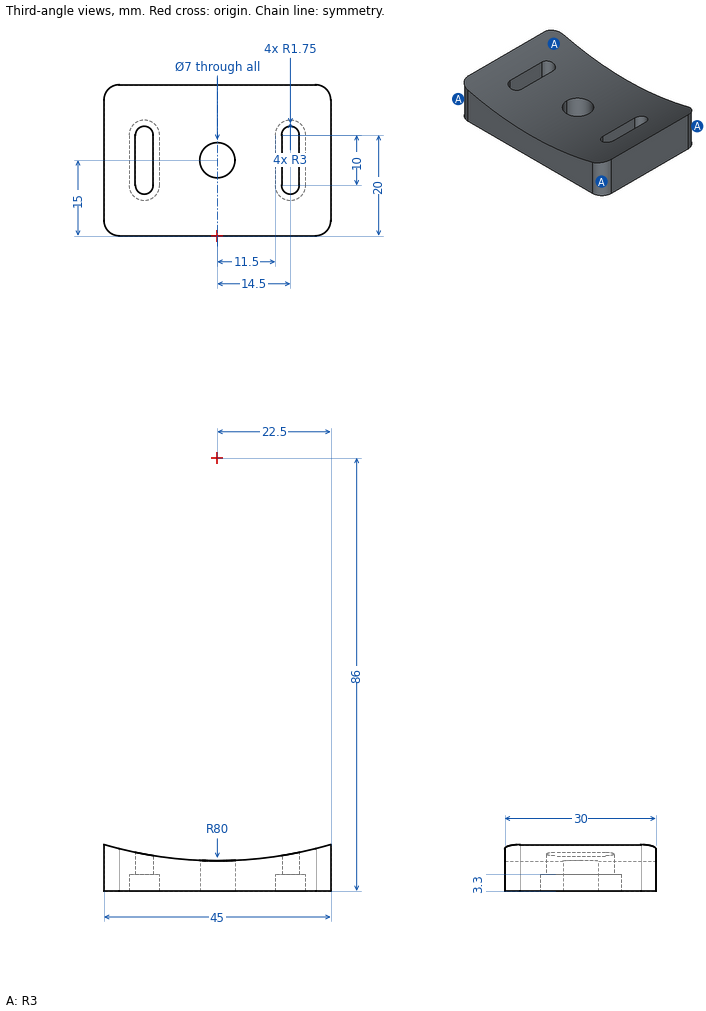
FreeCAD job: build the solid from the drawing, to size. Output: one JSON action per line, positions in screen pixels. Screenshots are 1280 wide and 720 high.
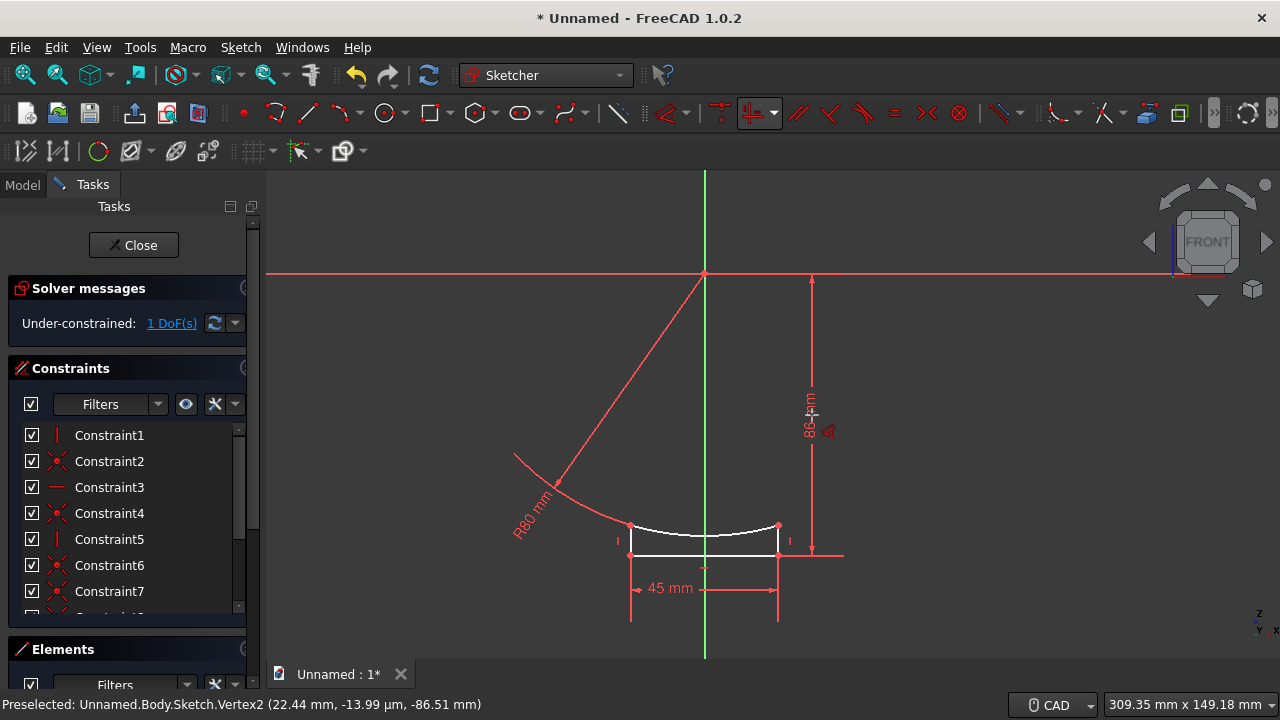
{"action": "left_click", "coordinate": [778, 525]}
{"action": "left_click", "coordinate": [742, 240]}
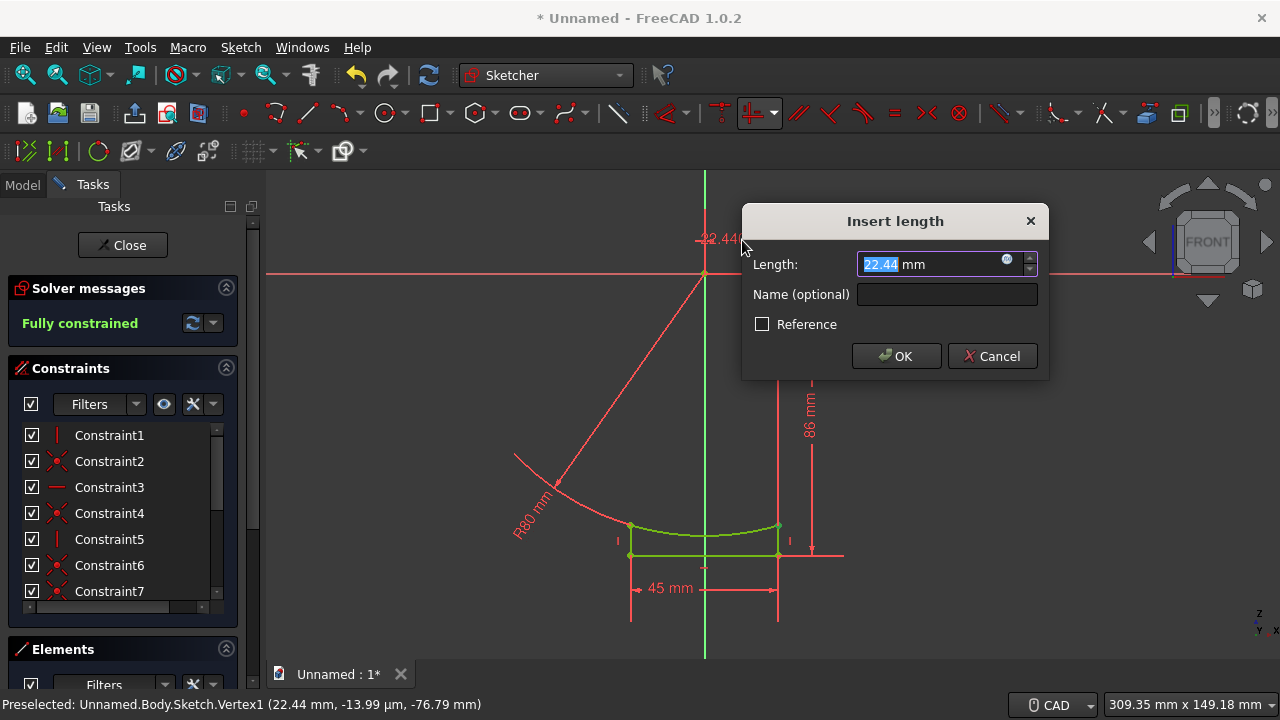
{"action": "type", "text": "22.5"}
{"action": "key", "text": "Return"}
{"action": "key", "text": "Escape"}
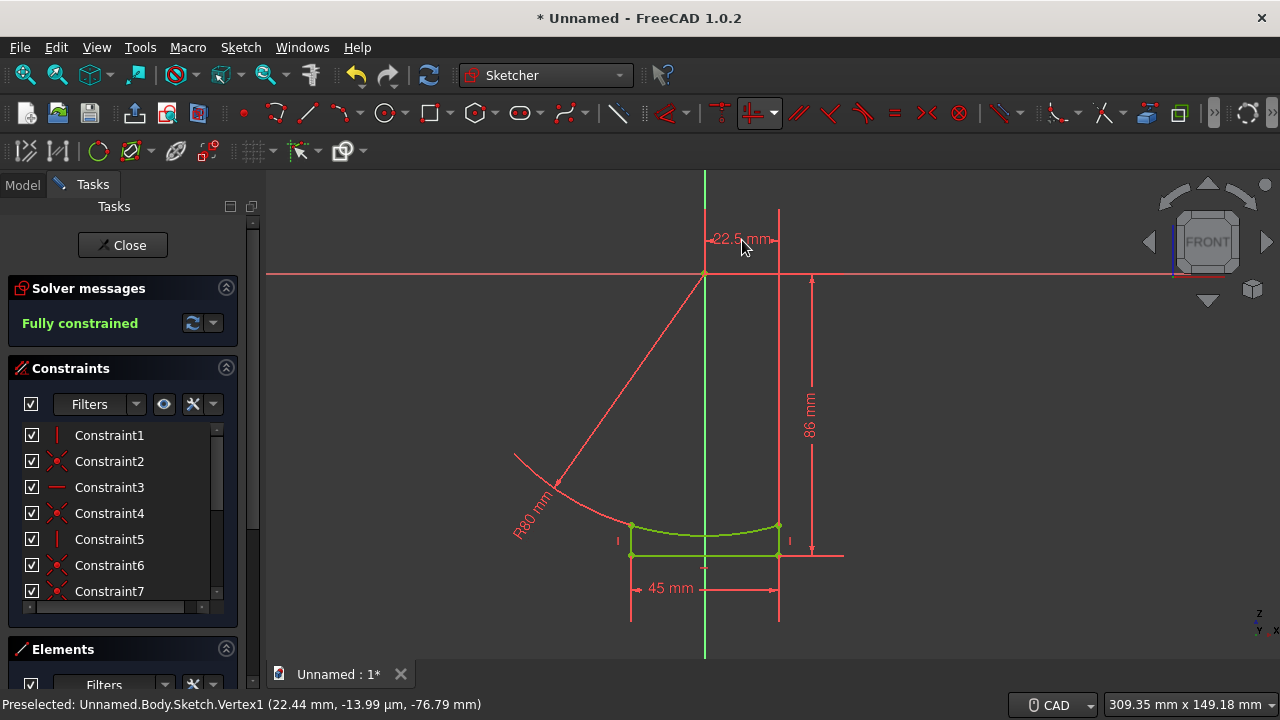
{"action": "left_click", "coordinate": [123, 245]}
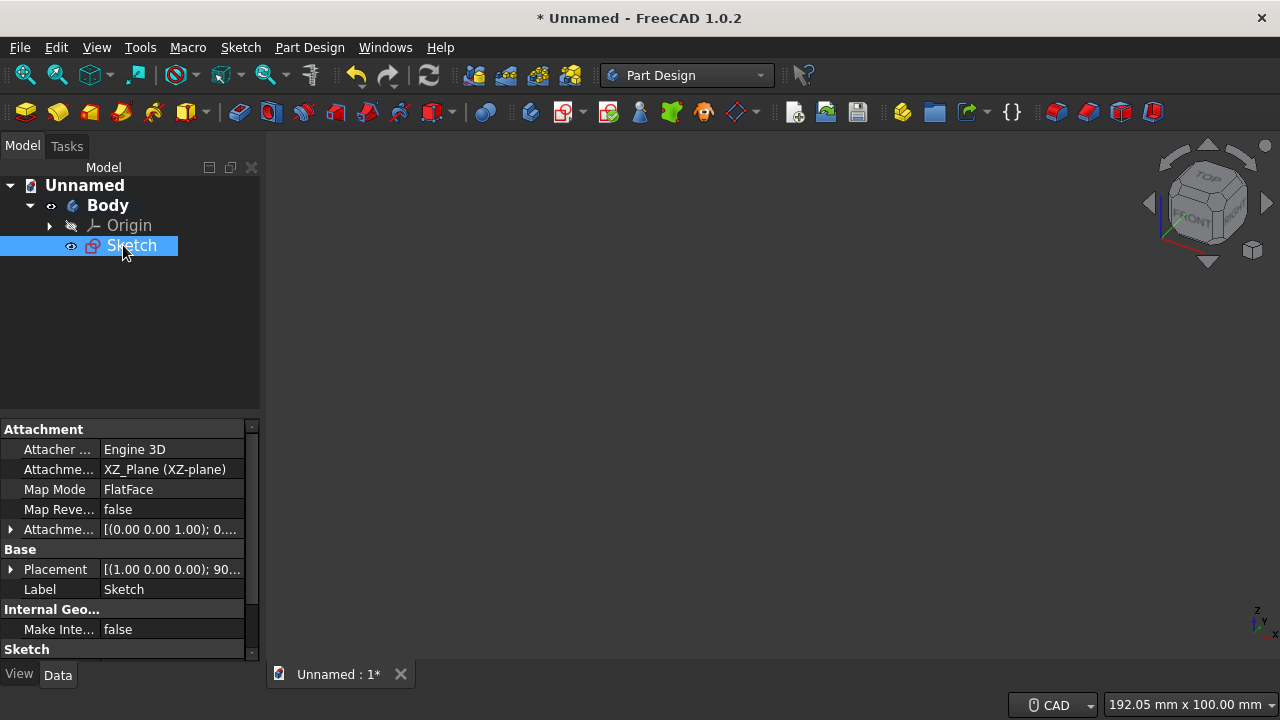
{"action": "left_click", "coordinate": [26, 112]}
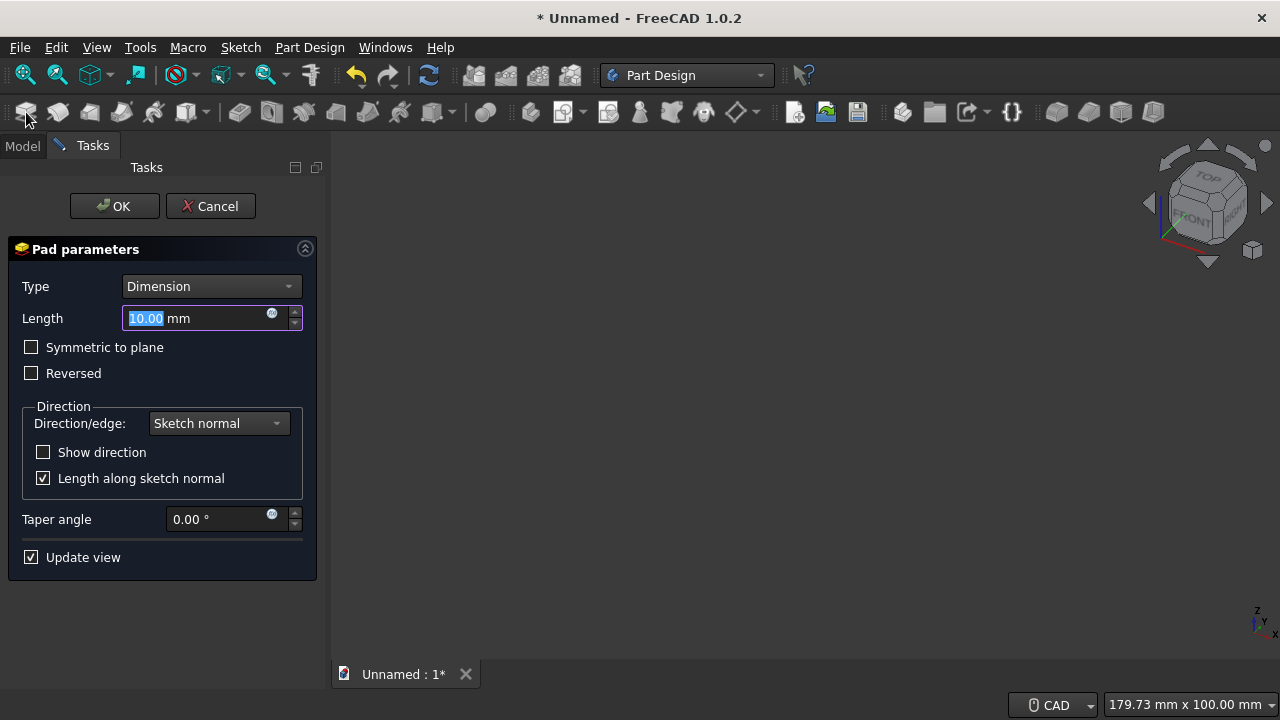
{"action": "type", "text": "30"}
{"action": "key", "text": "Tab"}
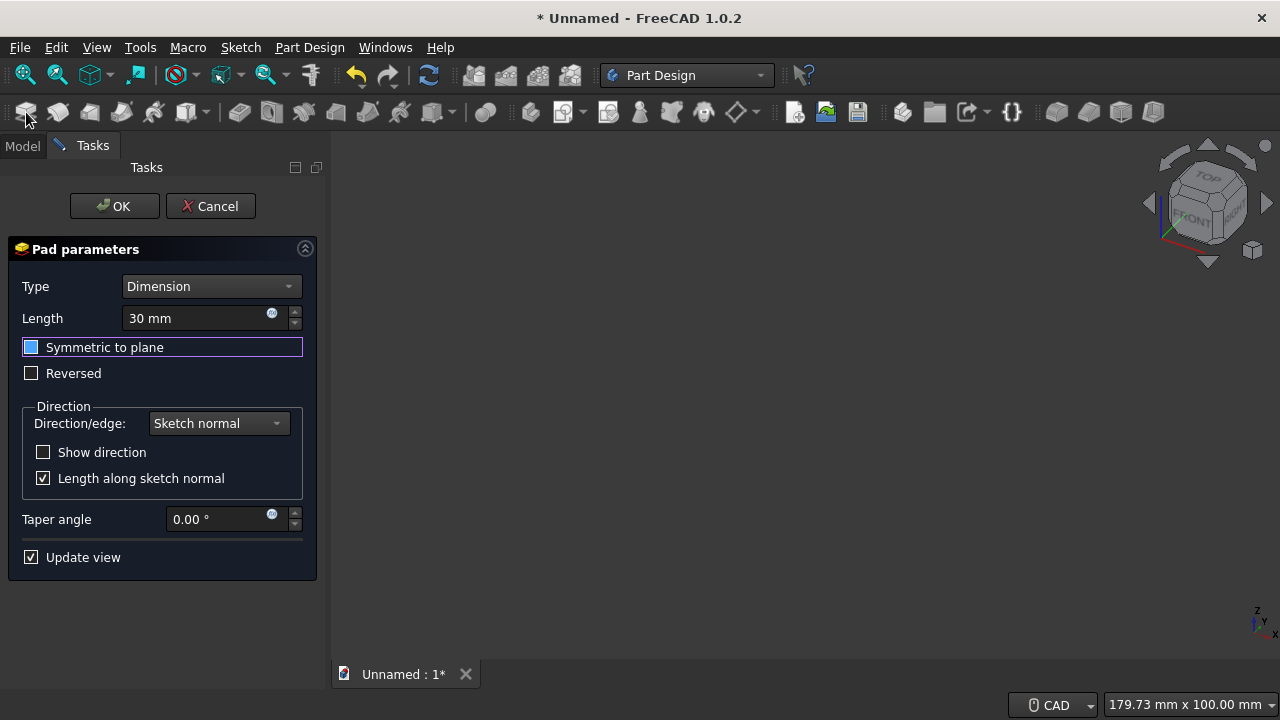
{"action": "left_click", "coordinate": [30, 373]}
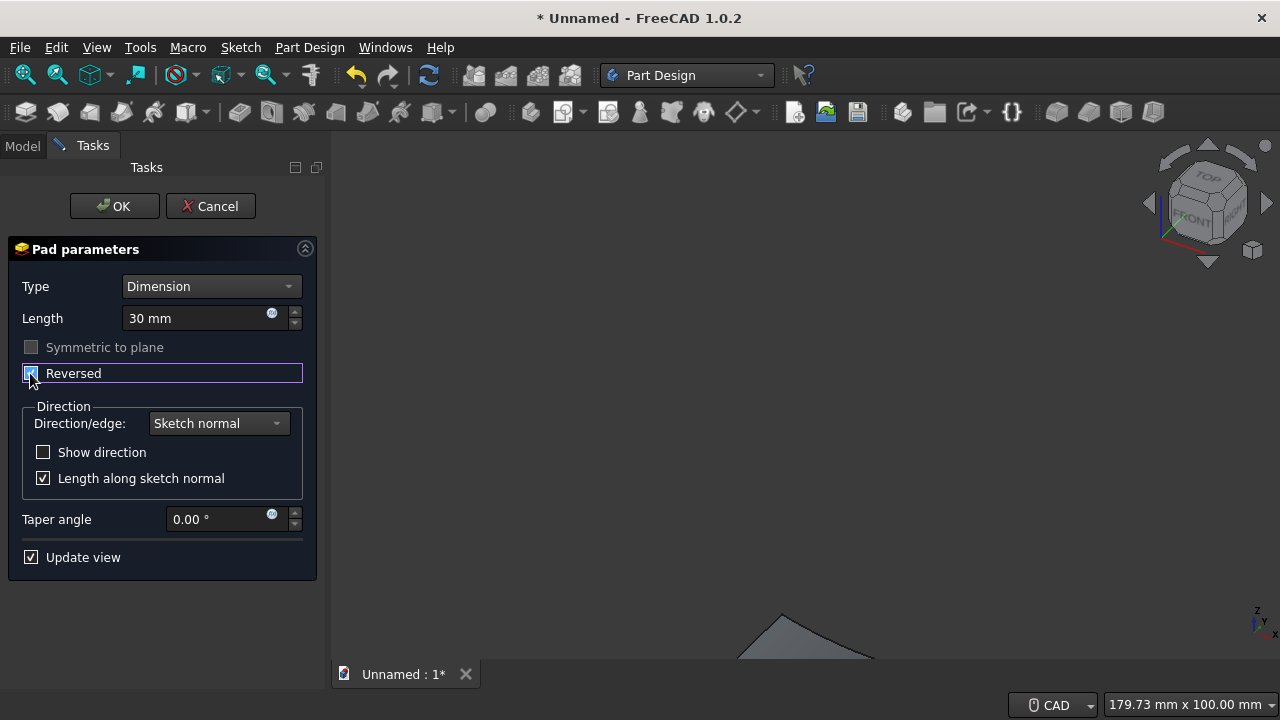
{"action": "left_click", "coordinate": [115, 206]}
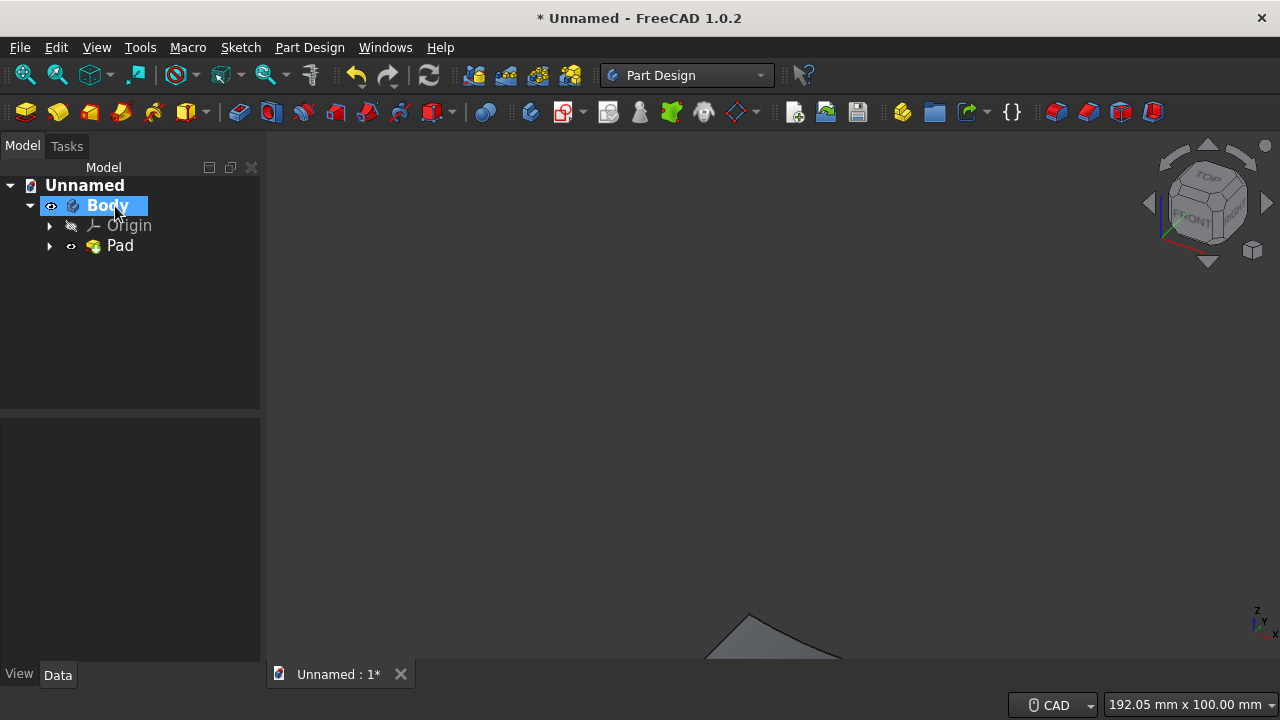
{"action": "key", "text": "v f"}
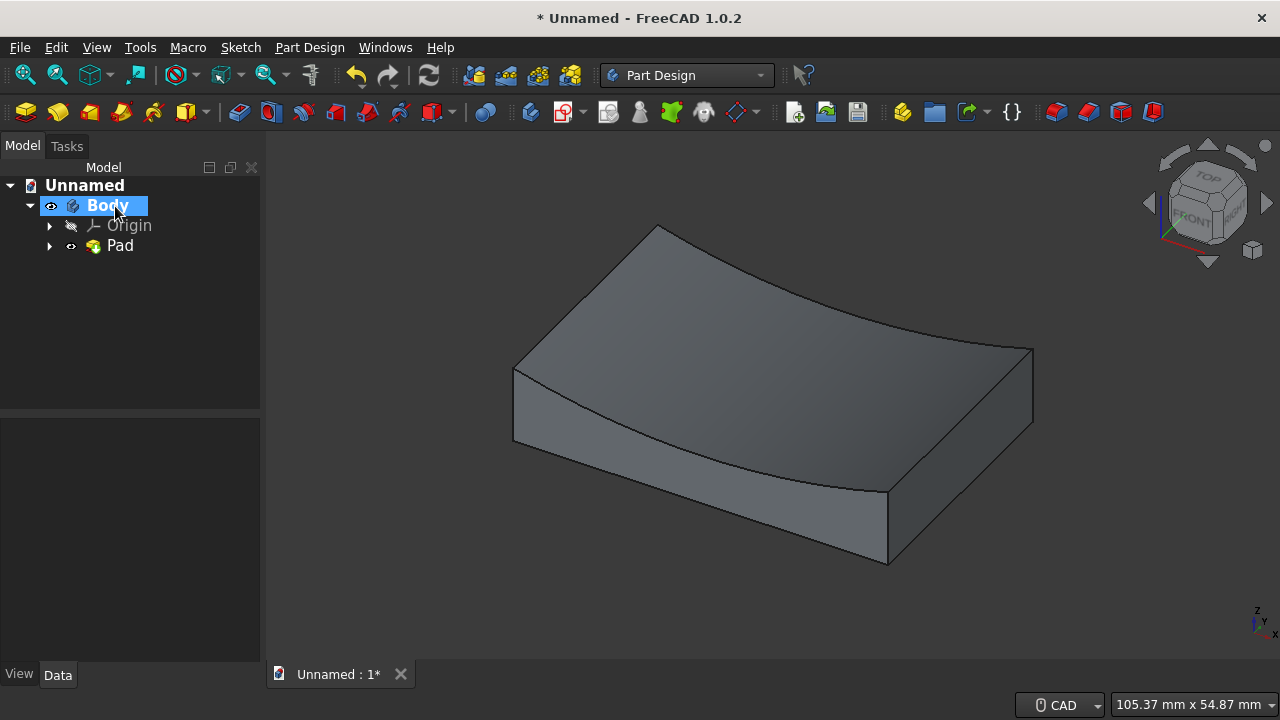
{"action": "left_click", "coordinate": [888, 528]}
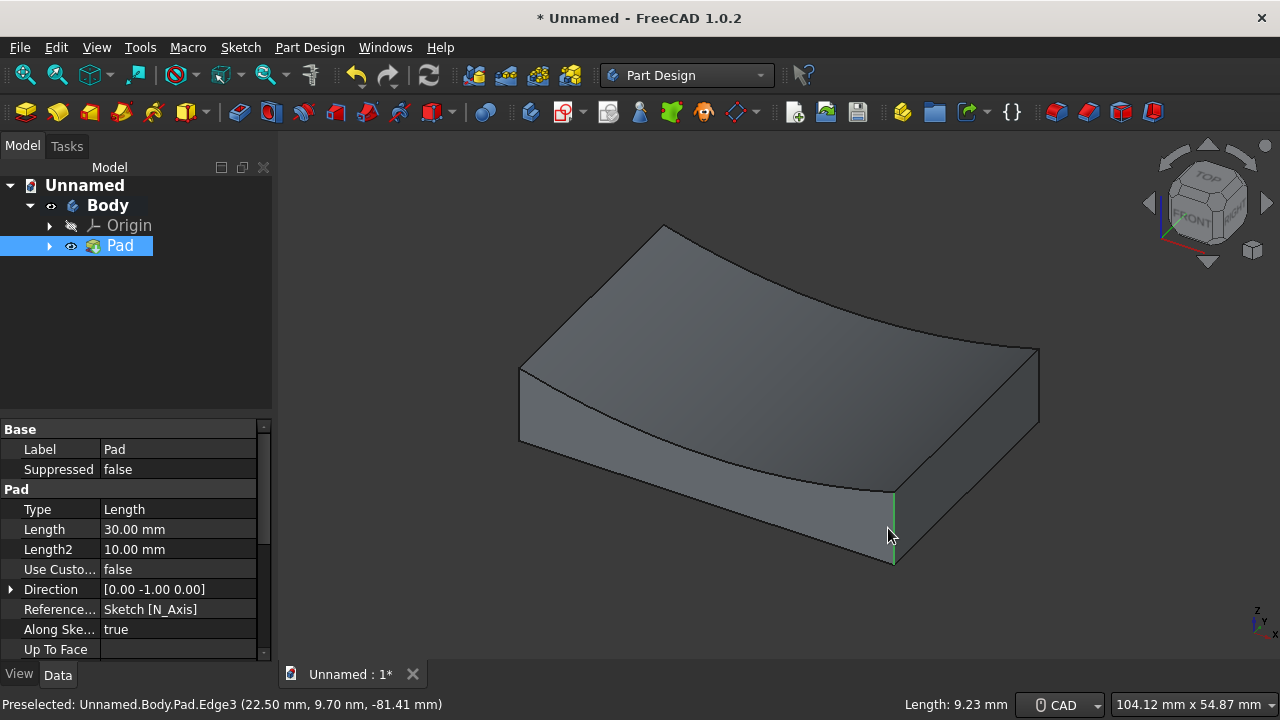
{"action": "key", "text": "0"}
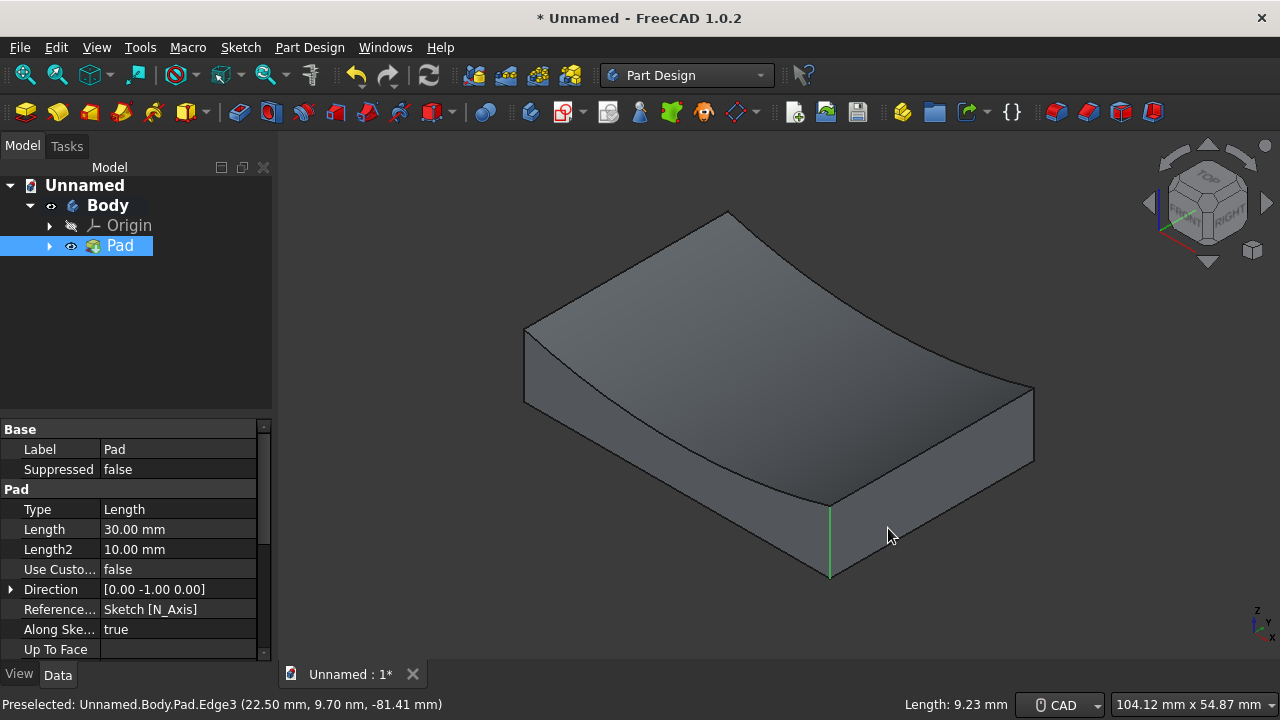
{"action": "key", "text": "2"}